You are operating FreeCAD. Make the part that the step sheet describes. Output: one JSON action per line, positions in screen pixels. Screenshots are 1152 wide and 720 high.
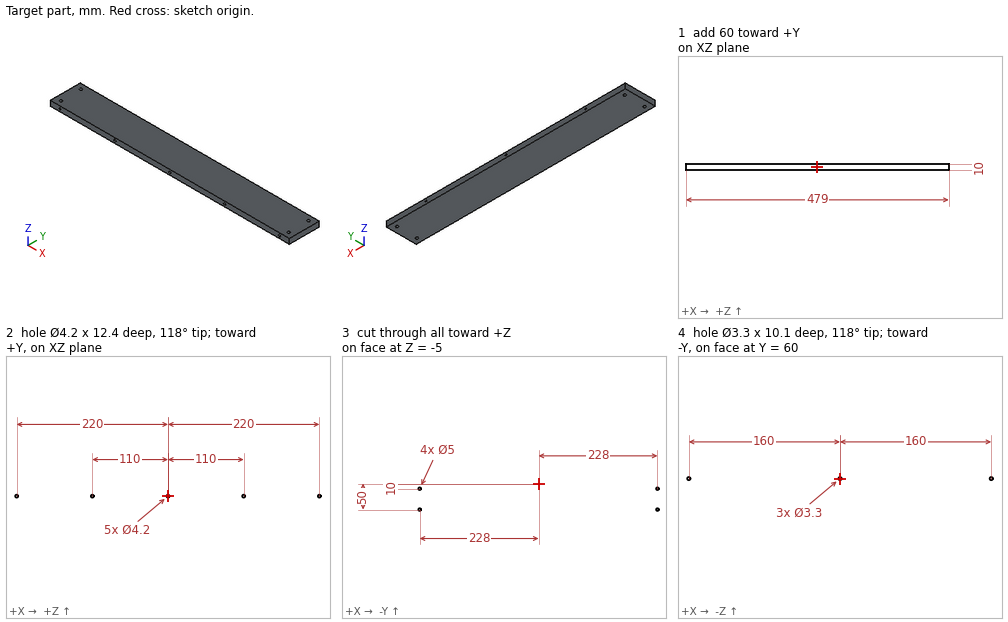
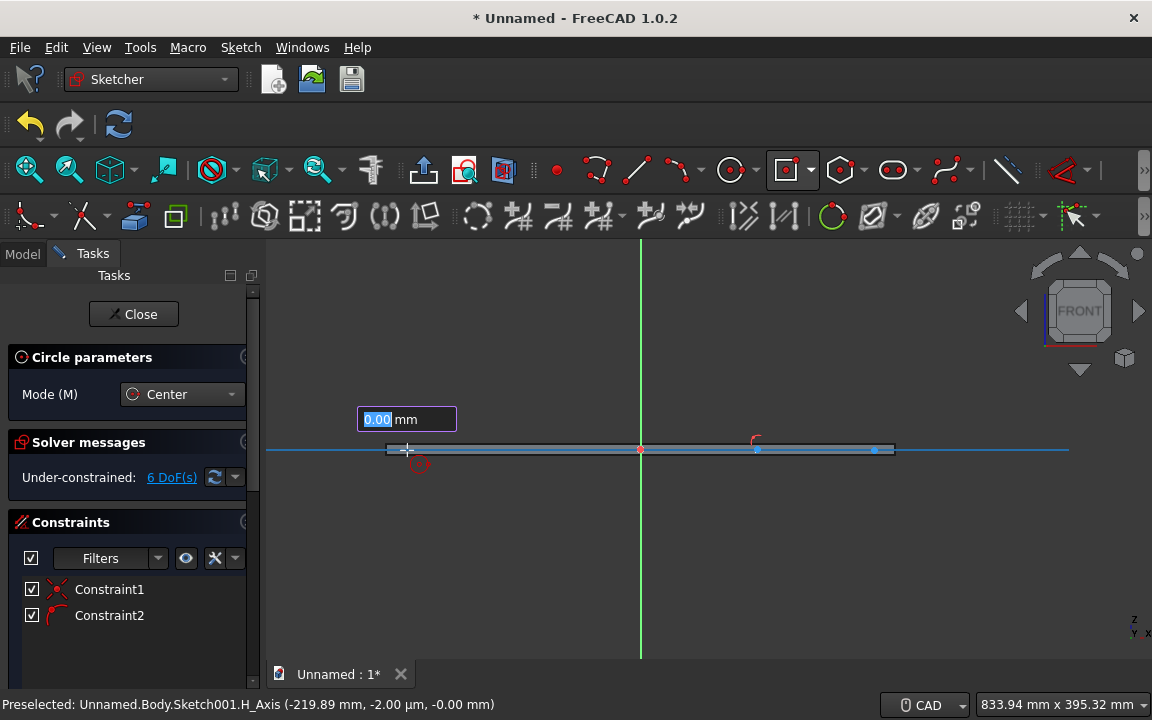
{"action": "scroll", "coordinate": [408, 448], "scroll_direction": "up", "scroll_amount": 11}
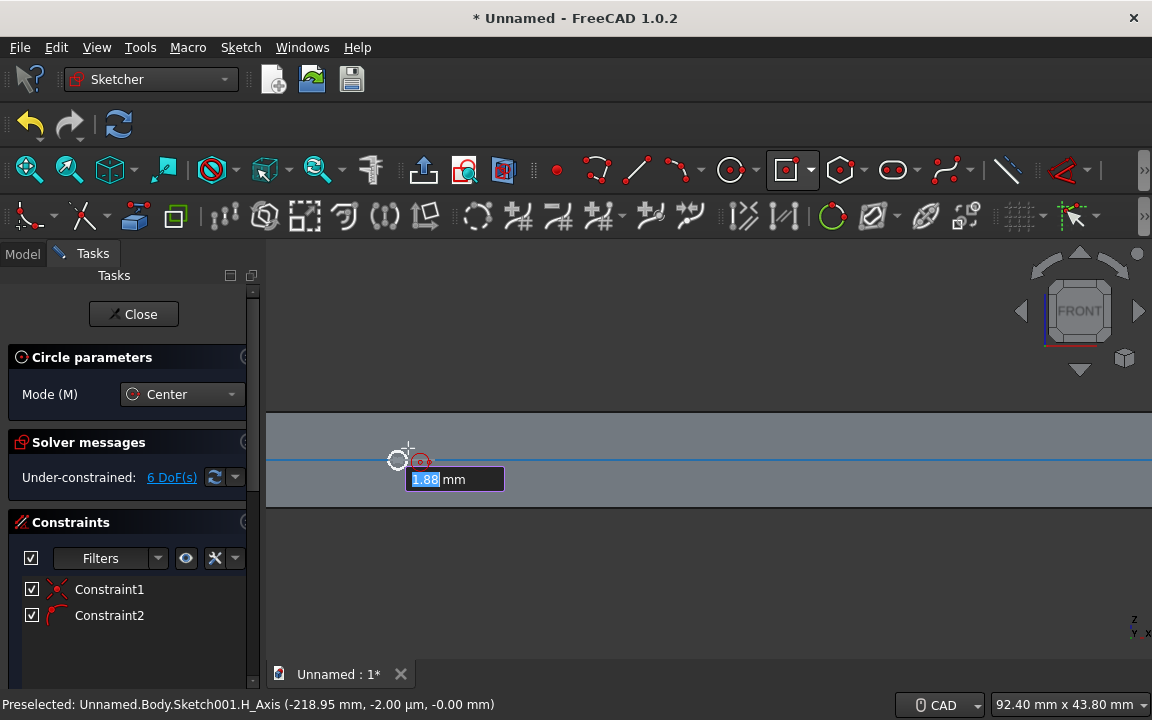
{"action": "left_click", "coordinate": [404, 441]}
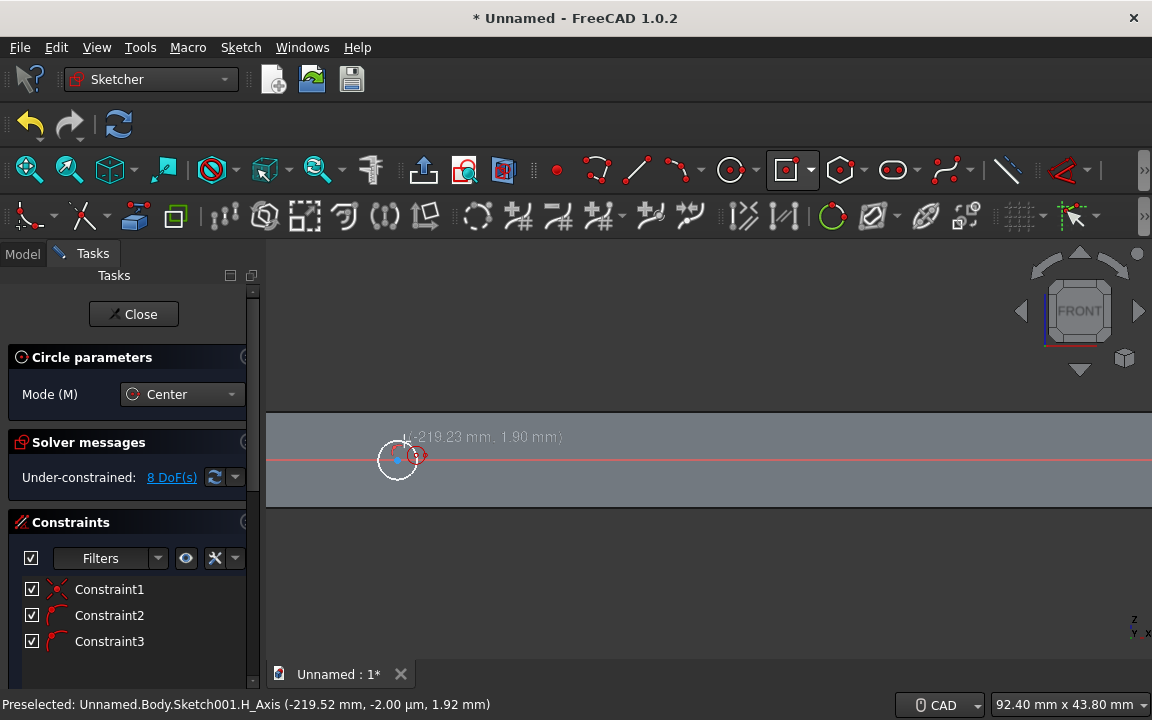
{"action": "scroll", "coordinate": [408, 448], "scroll_direction": "down", "scroll_amount": 11}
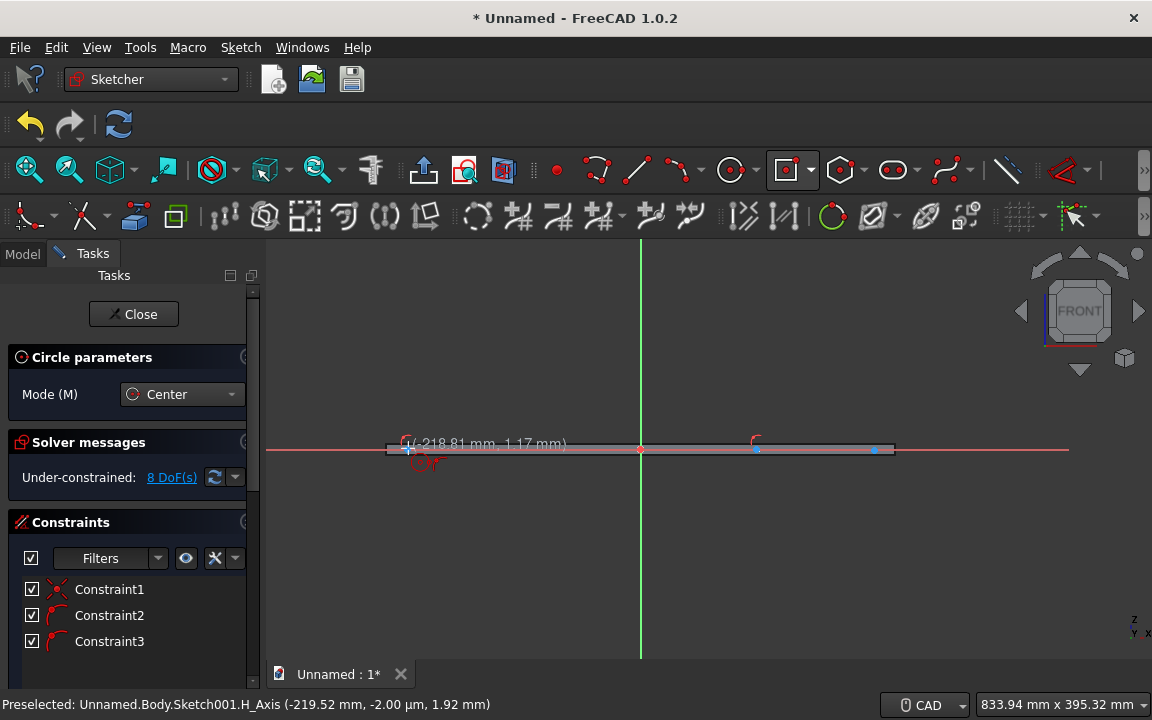
{"action": "scroll", "coordinate": [524, 450], "scroll_direction": "up", "scroll_amount": 12}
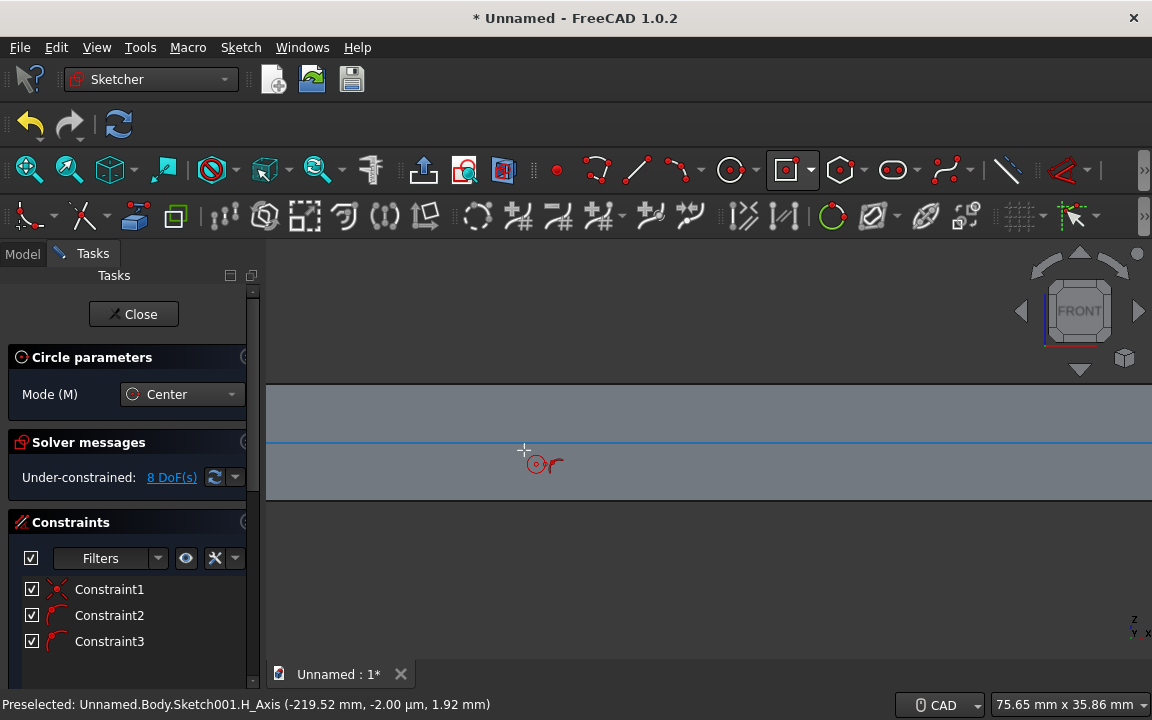
{"action": "scroll", "coordinate": [524, 450], "scroll_direction": "down", "scroll_amount": 12}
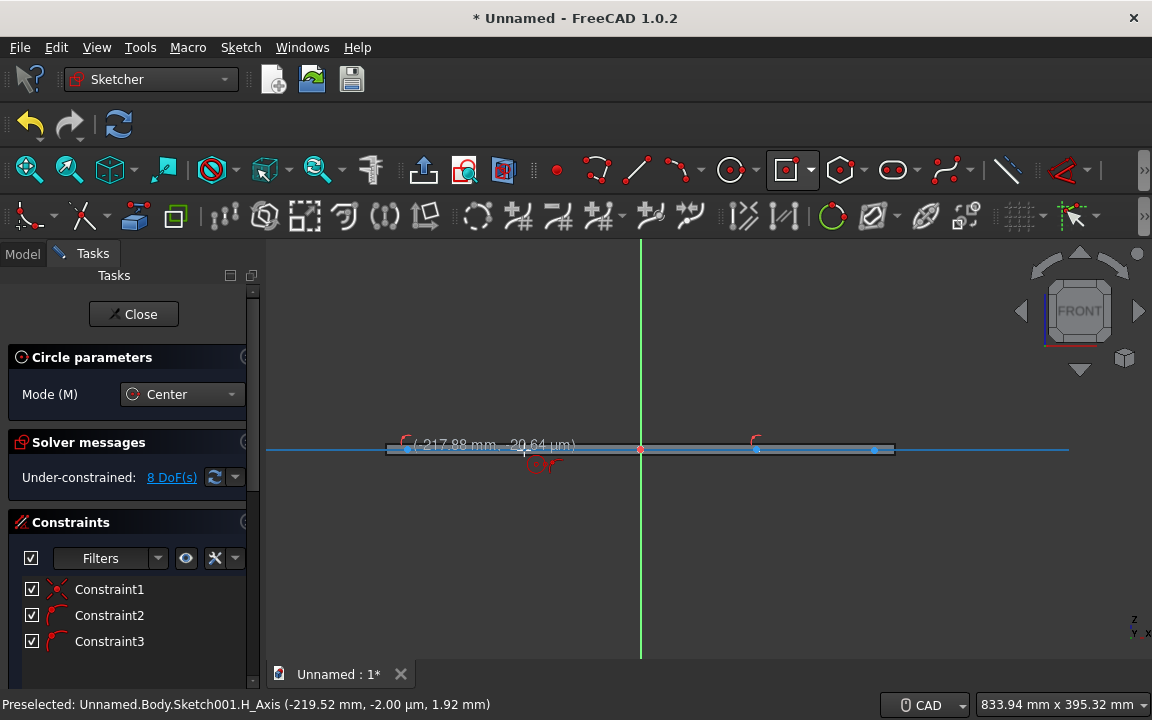
{"action": "left_click", "coordinate": [524, 450]}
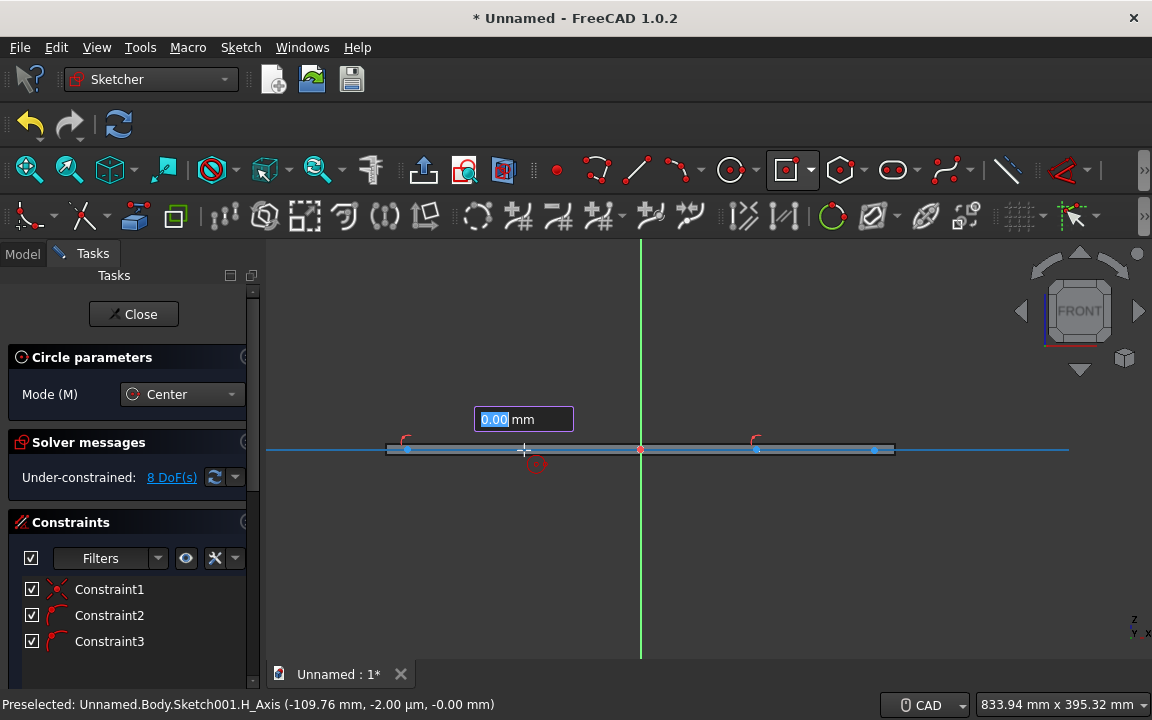
{"action": "scroll", "coordinate": [525, 448], "scroll_direction": "up", "scroll_amount": 11}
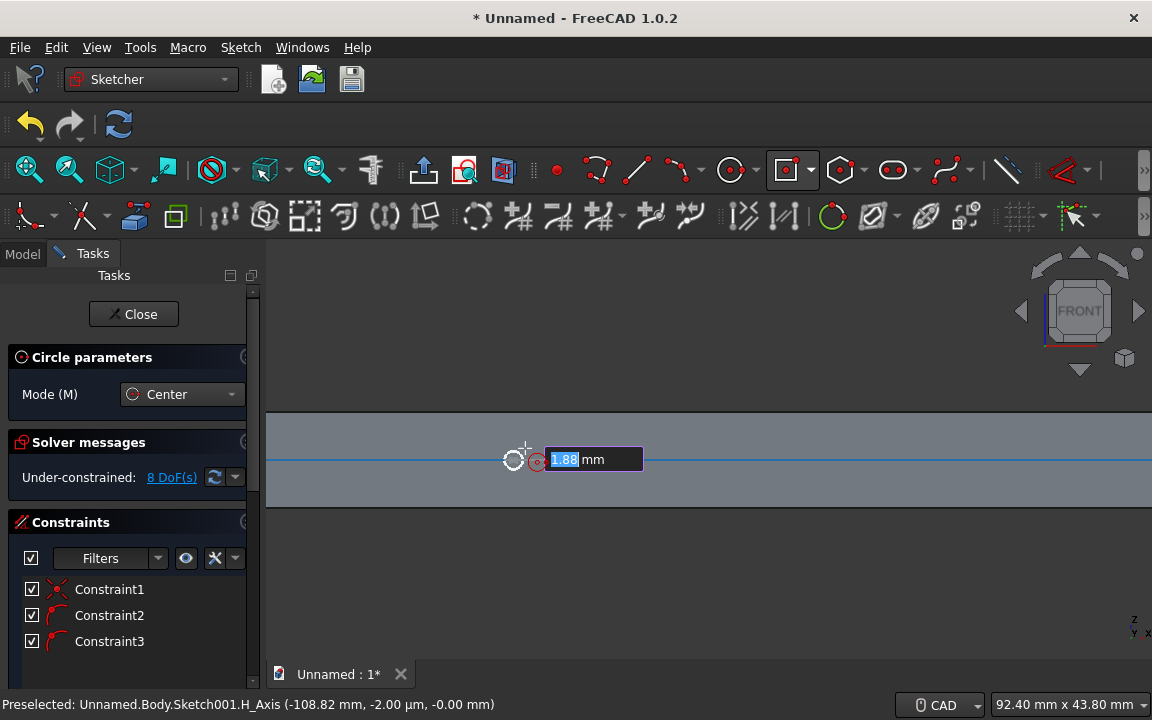
{"action": "left_click", "coordinate": [518, 441]}
{"action": "key", "text": "Escape"}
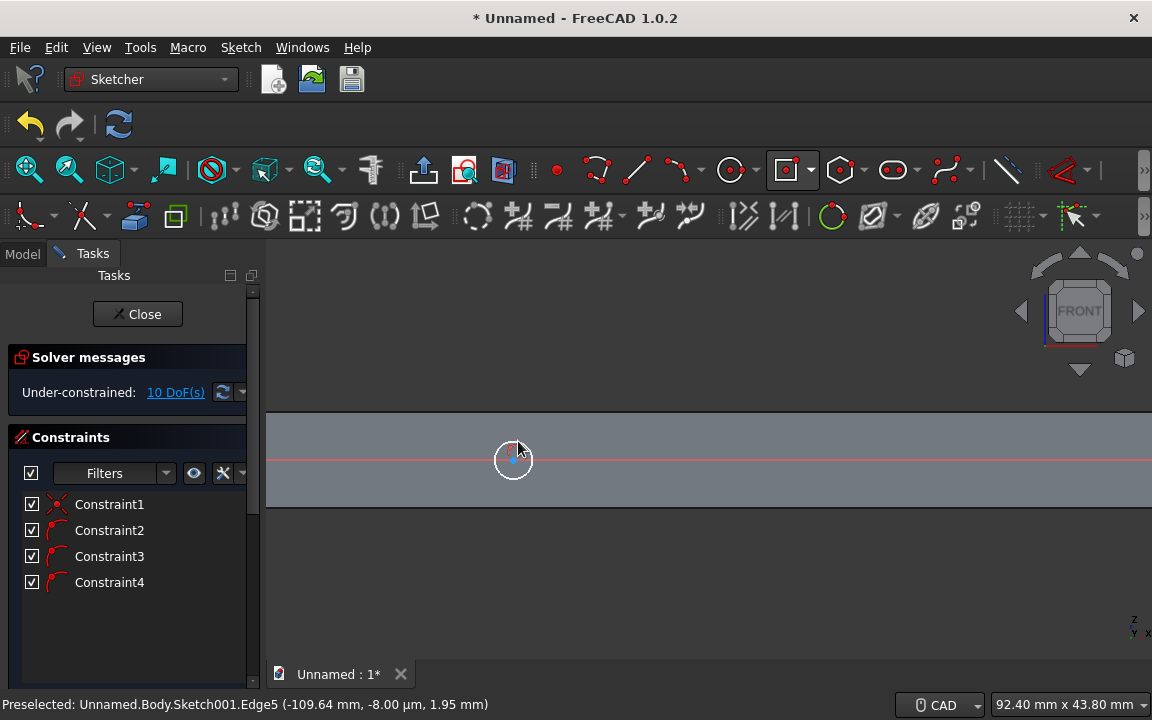
{"action": "scroll", "coordinate": [525, 448], "scroll_direction": "down", "scroll_amount": 11}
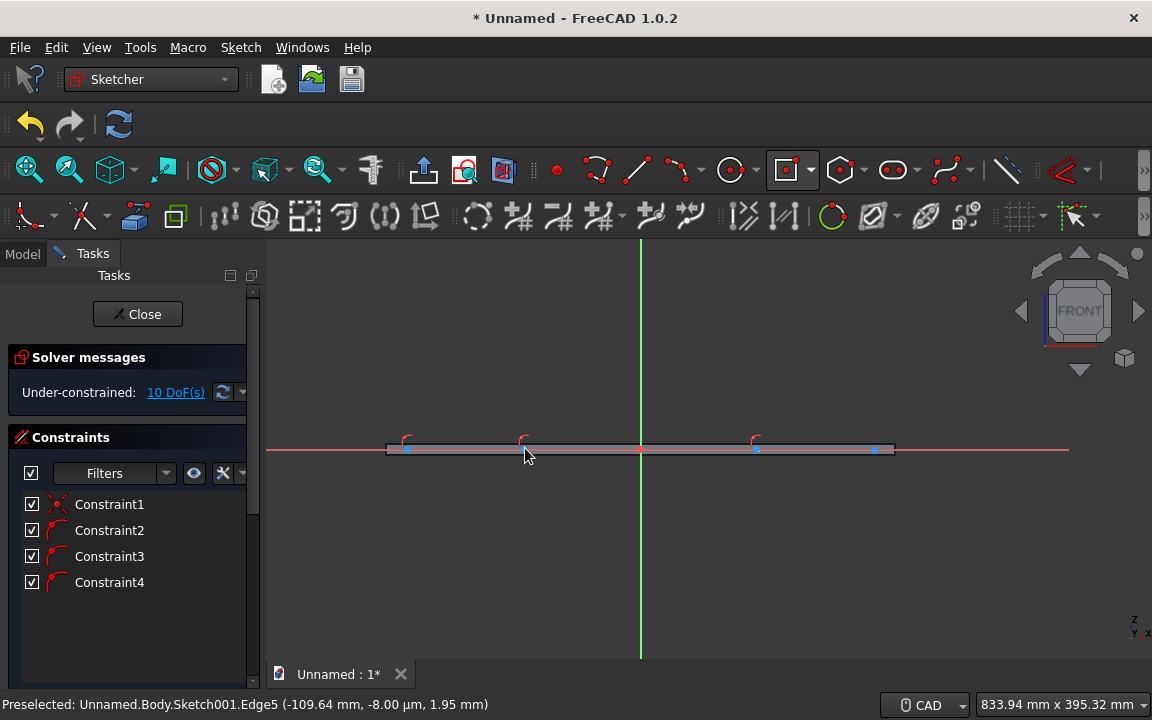
{"action": "scroll", "coordinate": [642, 448], "scroll_direction": "up", "scroll_amount": 11}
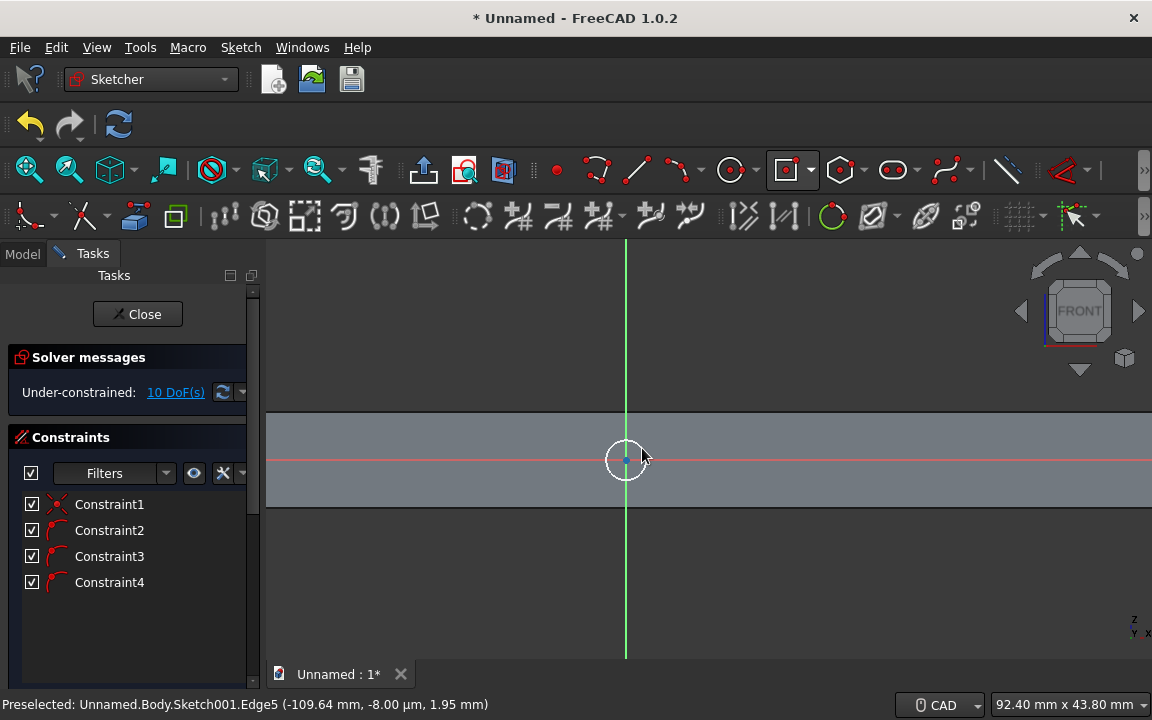
{"action": "left_click", "coordinate": [640, 446]}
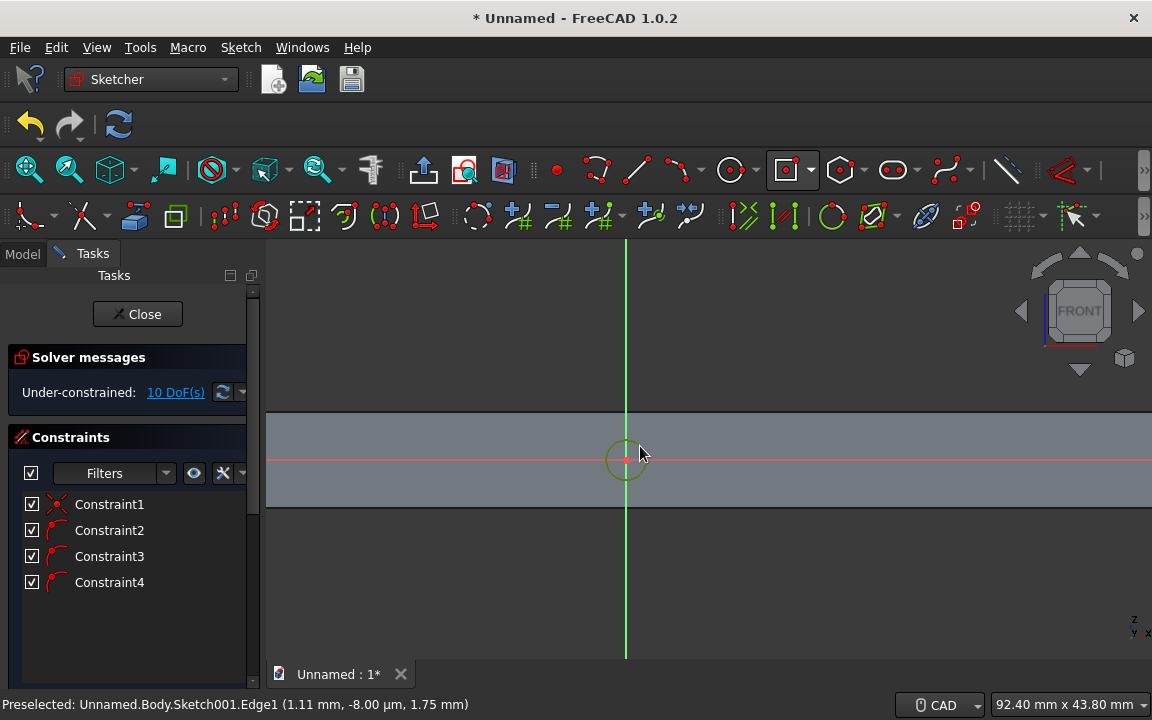
{"action": "scroll", "coordinate": [642, 448], "scroll_direction": "down", "scroll_amount": 11}